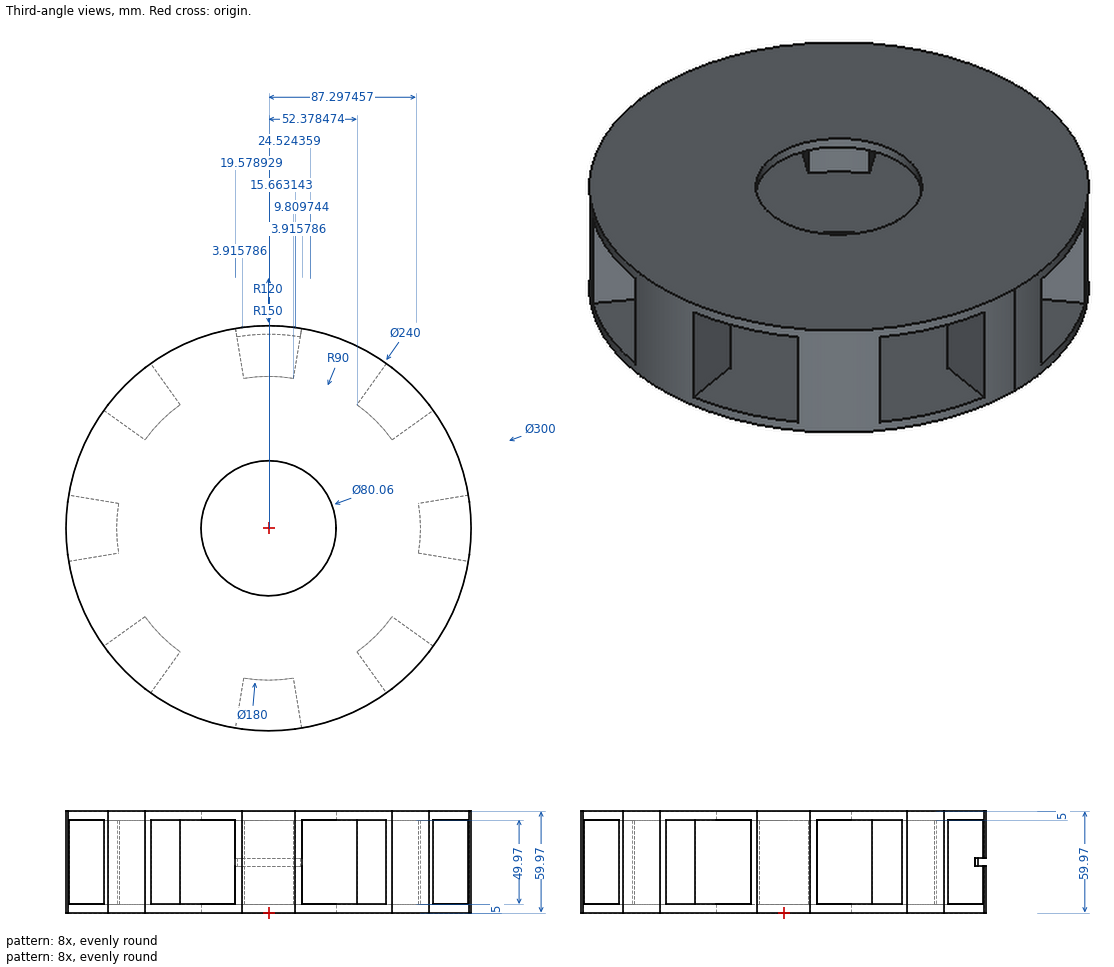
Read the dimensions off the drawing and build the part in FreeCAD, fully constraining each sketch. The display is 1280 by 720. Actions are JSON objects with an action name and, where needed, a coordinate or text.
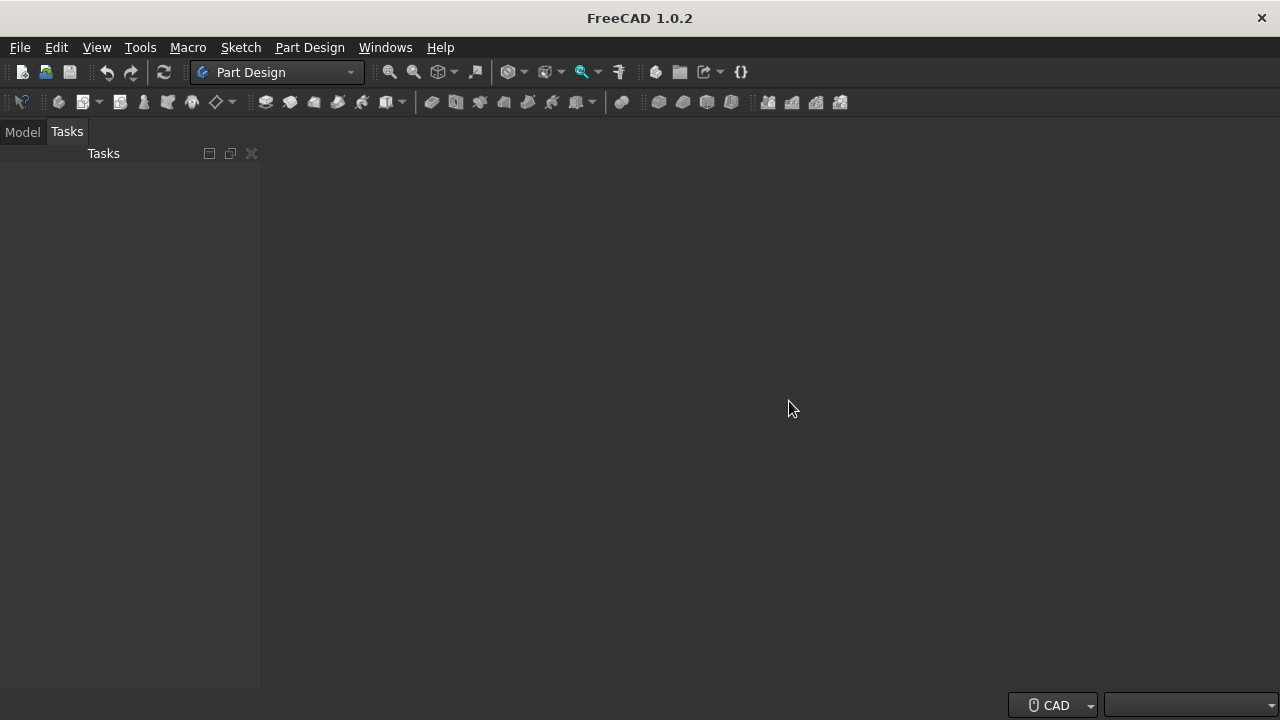
{"action": "left_click", "coordinate": [22, 72]}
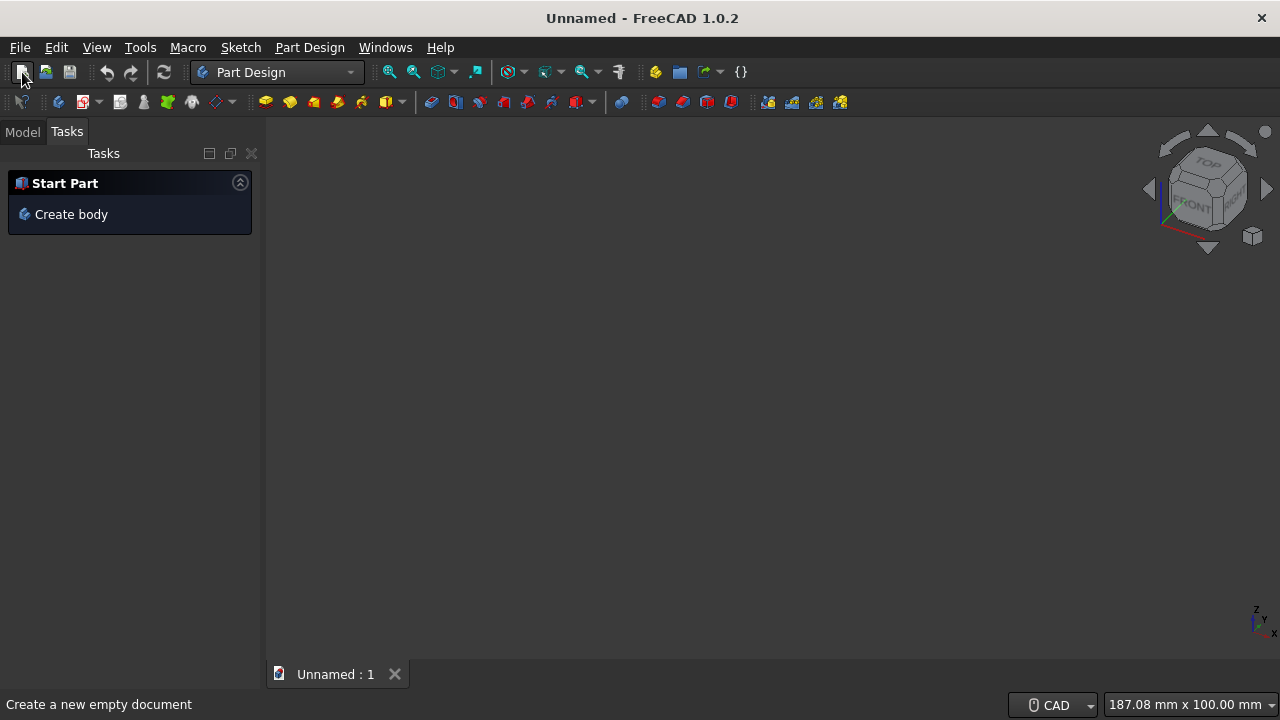
{"action": "left_click", "coordinate": [84, 102]}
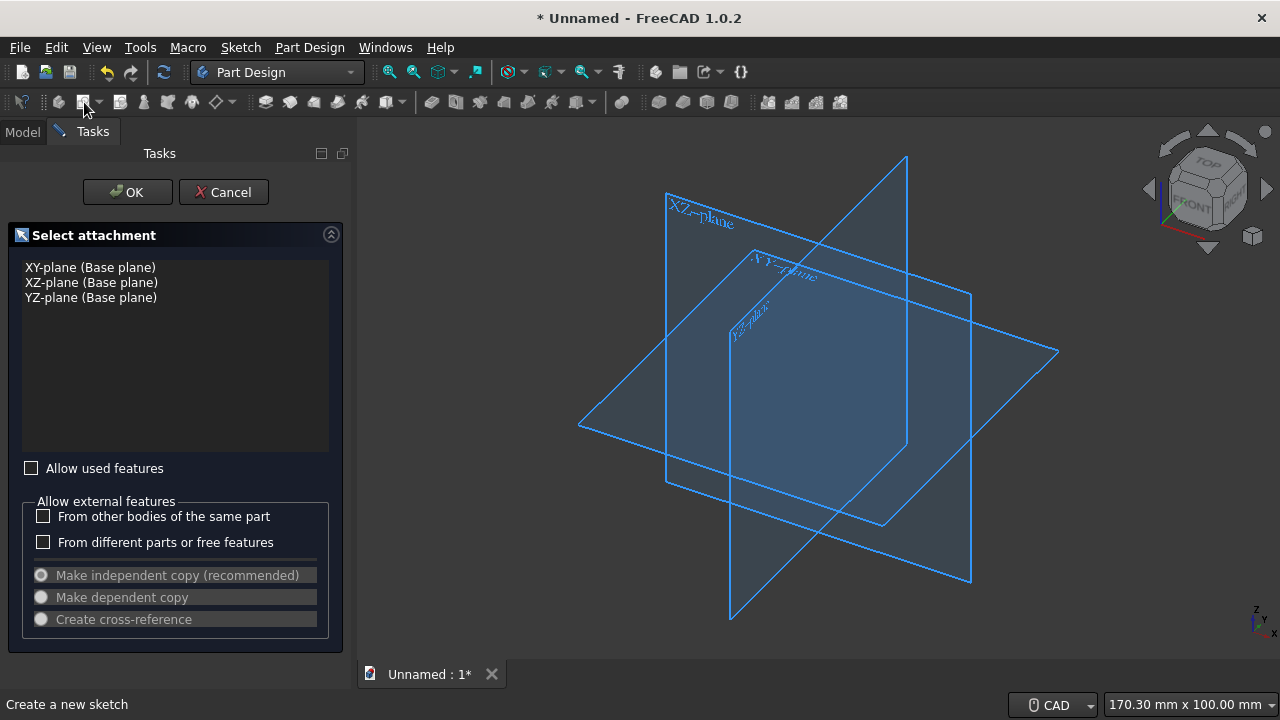
{"action": "left_click", "coordinate": [82, 268]}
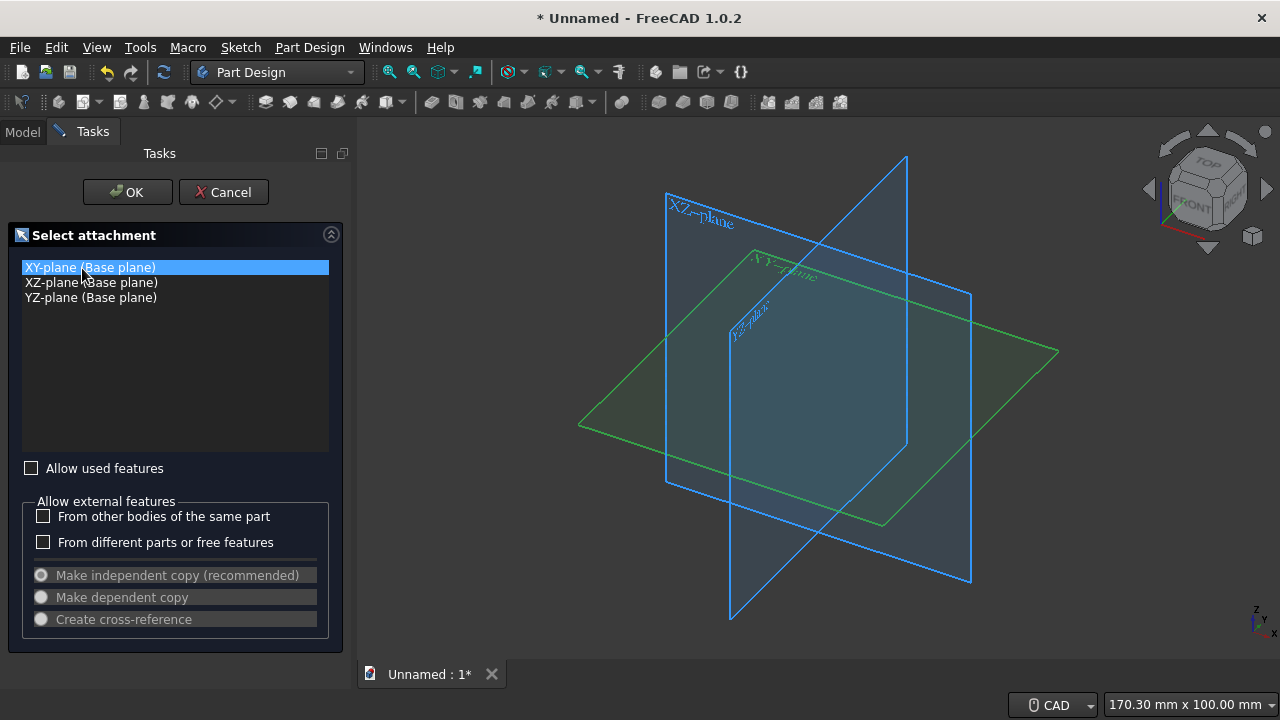
{"action": "left_click", "coordinate": [128, 192]}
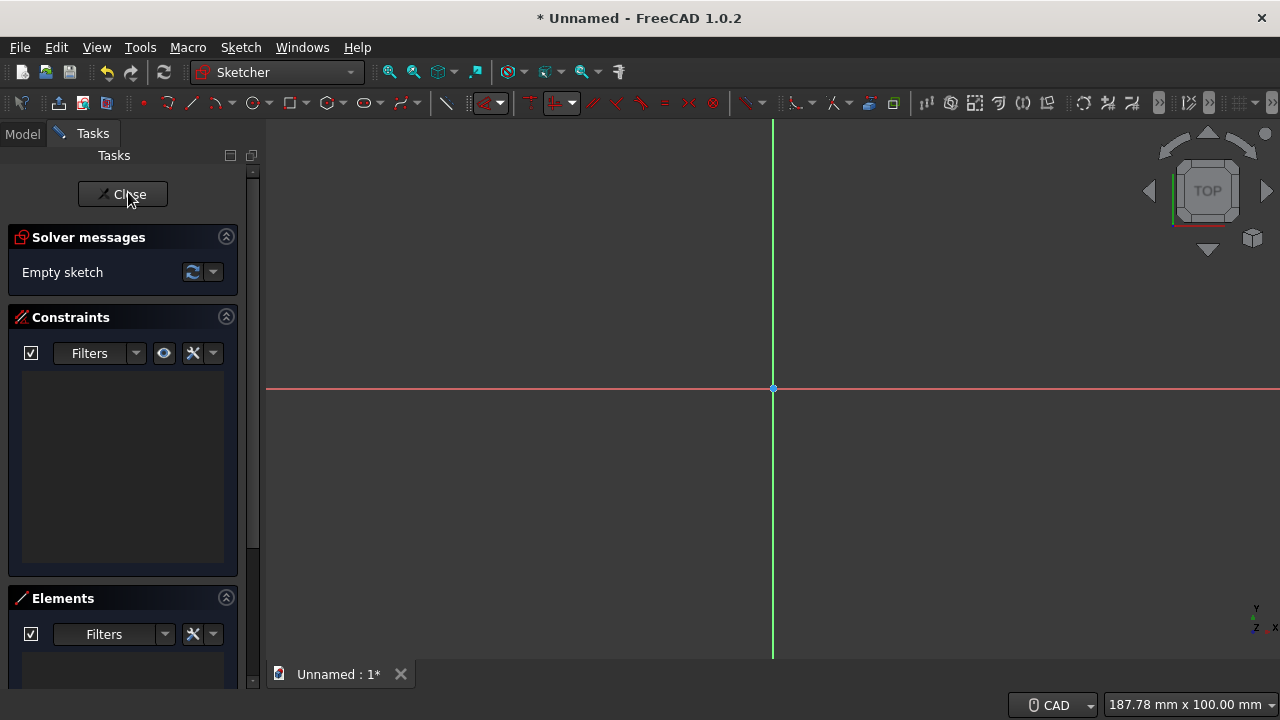
{"action": "scroll", "coordinate": [687, 389], "scroll_direction": "down", "scroll_amount": 8}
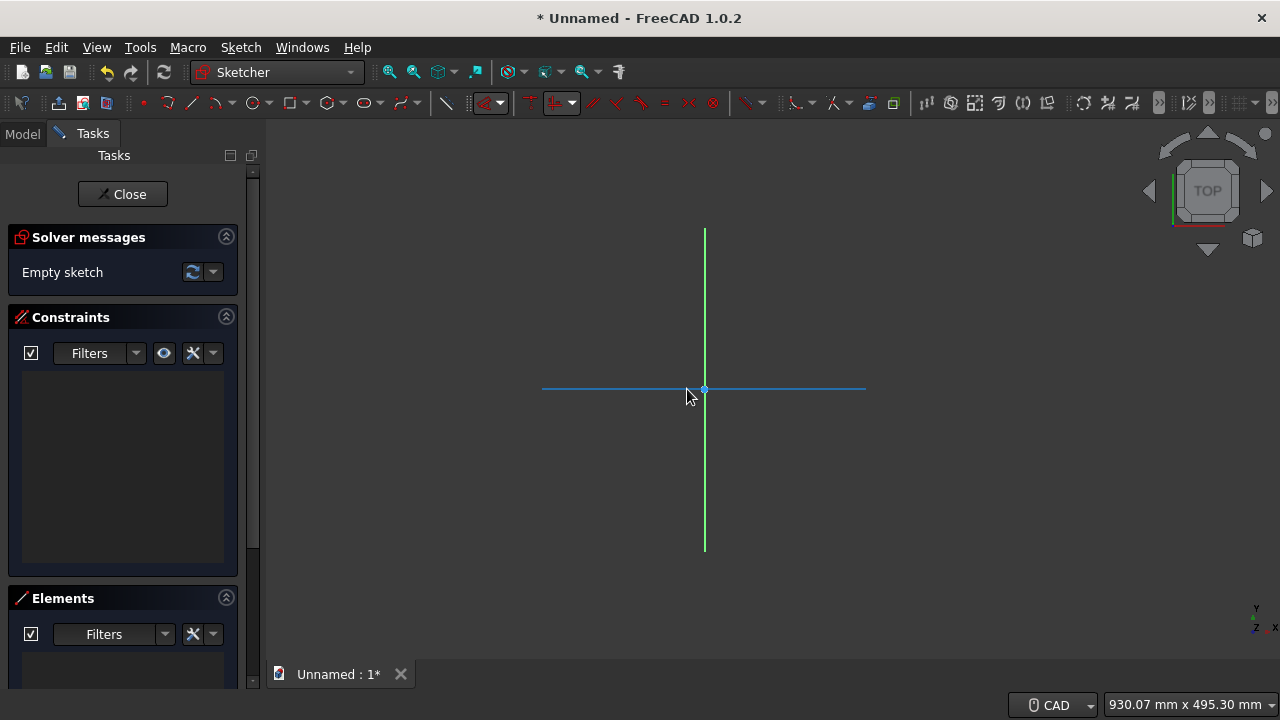
{"action": "left_click", "coordinate": [254, 104]}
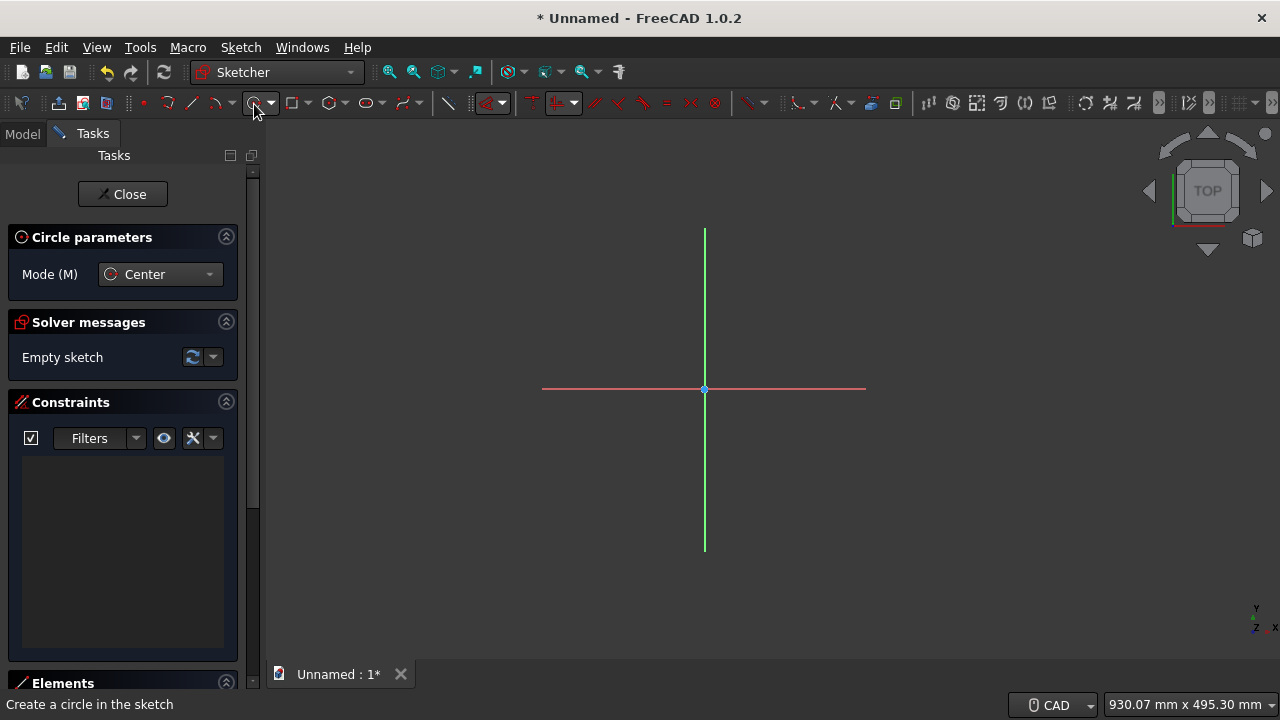
{"action": "left_click", "coordinate": [705, 389]}
{"action": "left_click", "coordinate": [820, 274]}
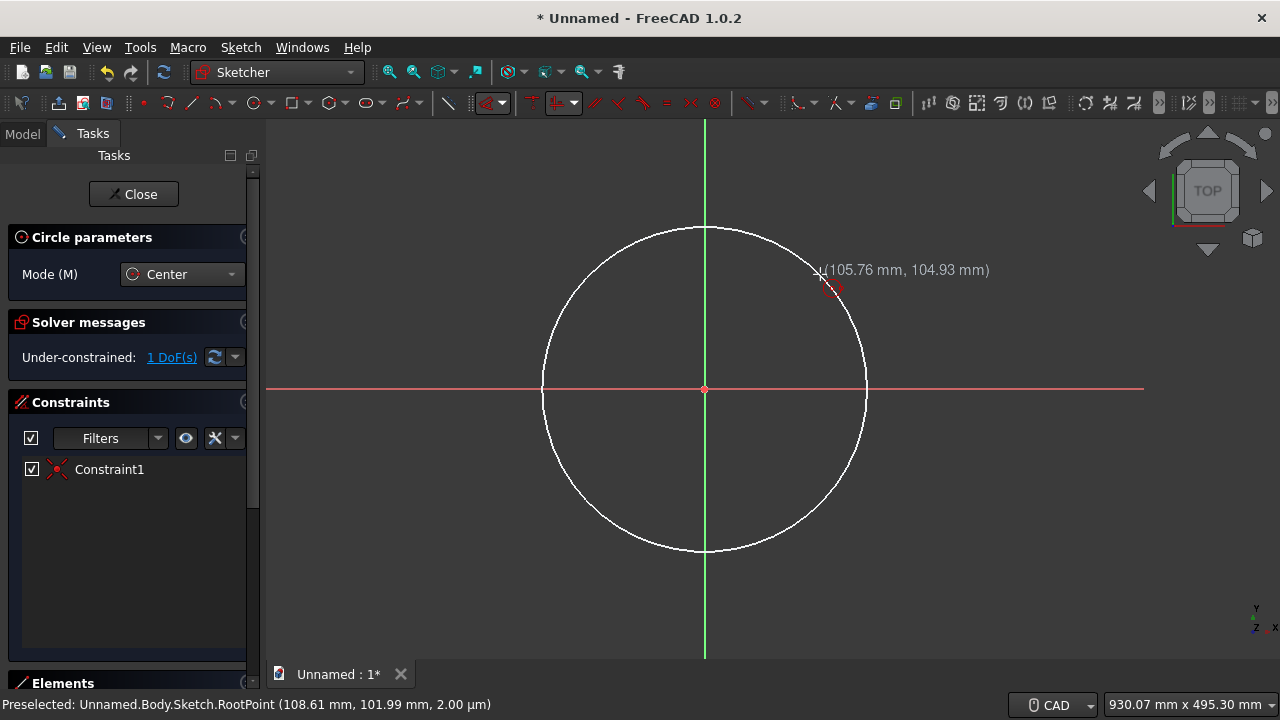
{"action": "left_click", "coordinate": [705, 389]}
{"action": "left_click", "coordinate": [797, 297]}
{"action": "key", "text": "Escape"}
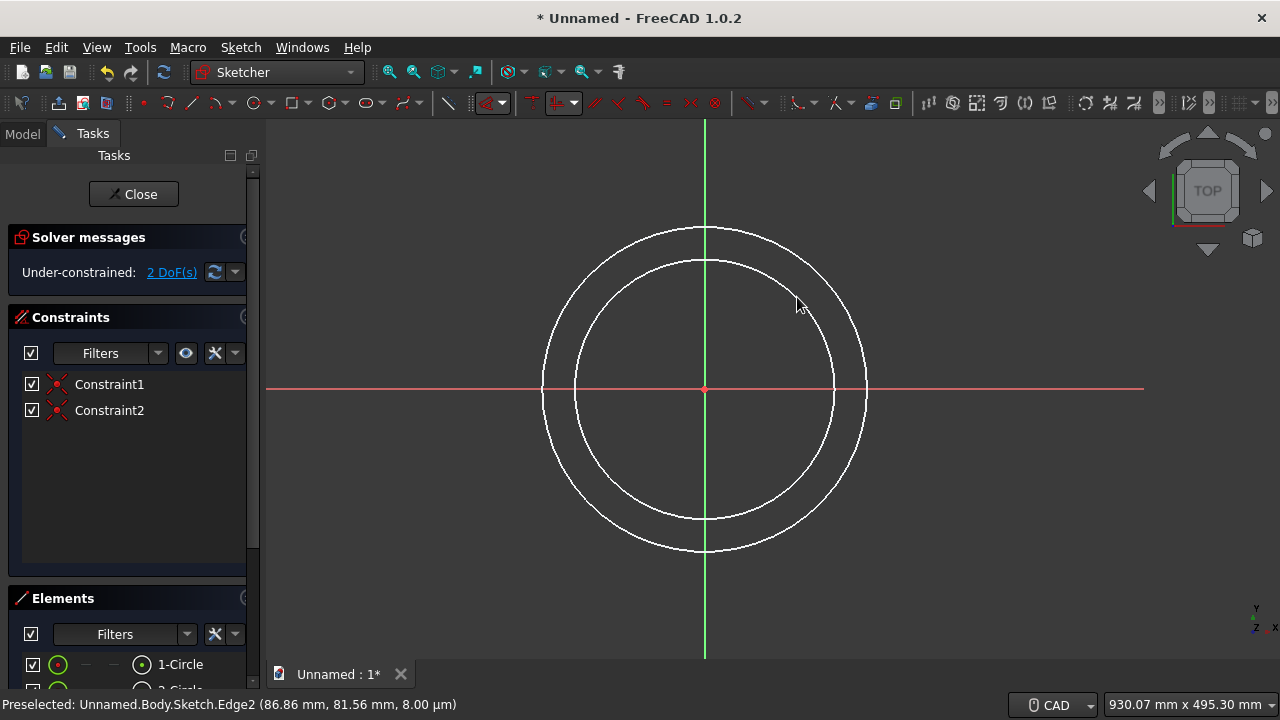
{"action": "key", "text": "d"}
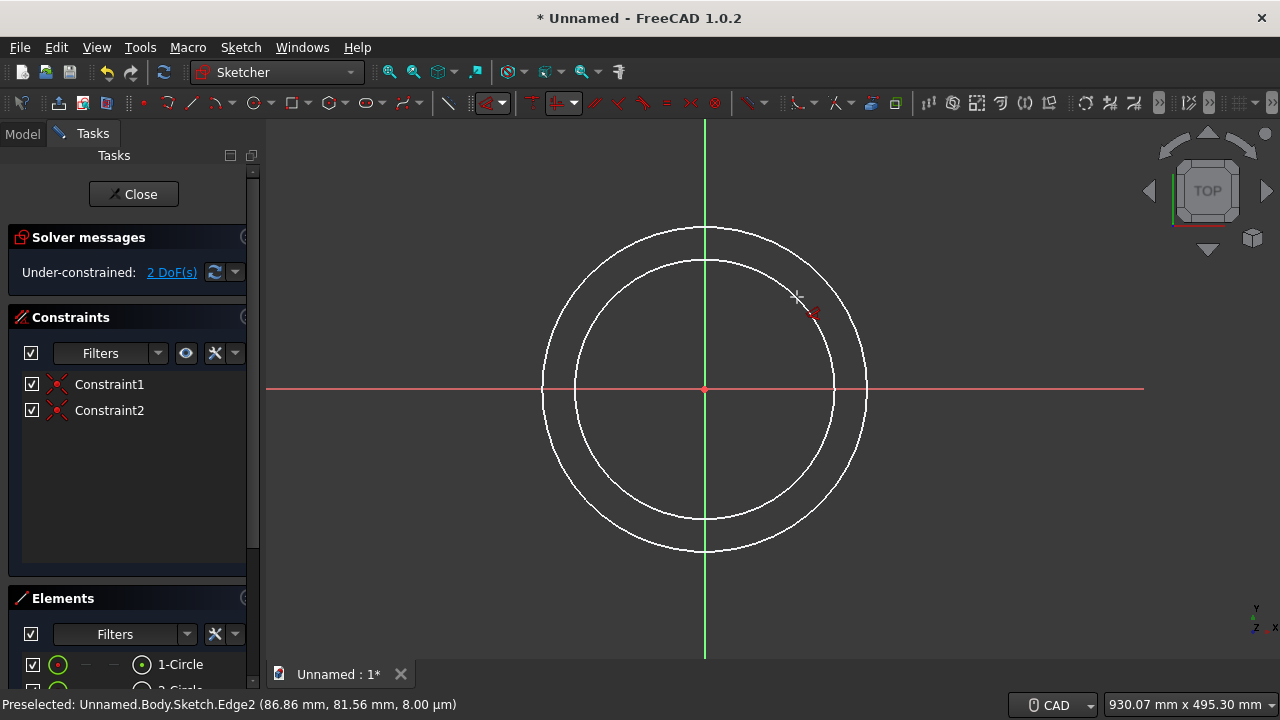
{"action": "left_click", "coordinate": [819, 274]}
{"action": "left_click", "coordinate": [842, 251]}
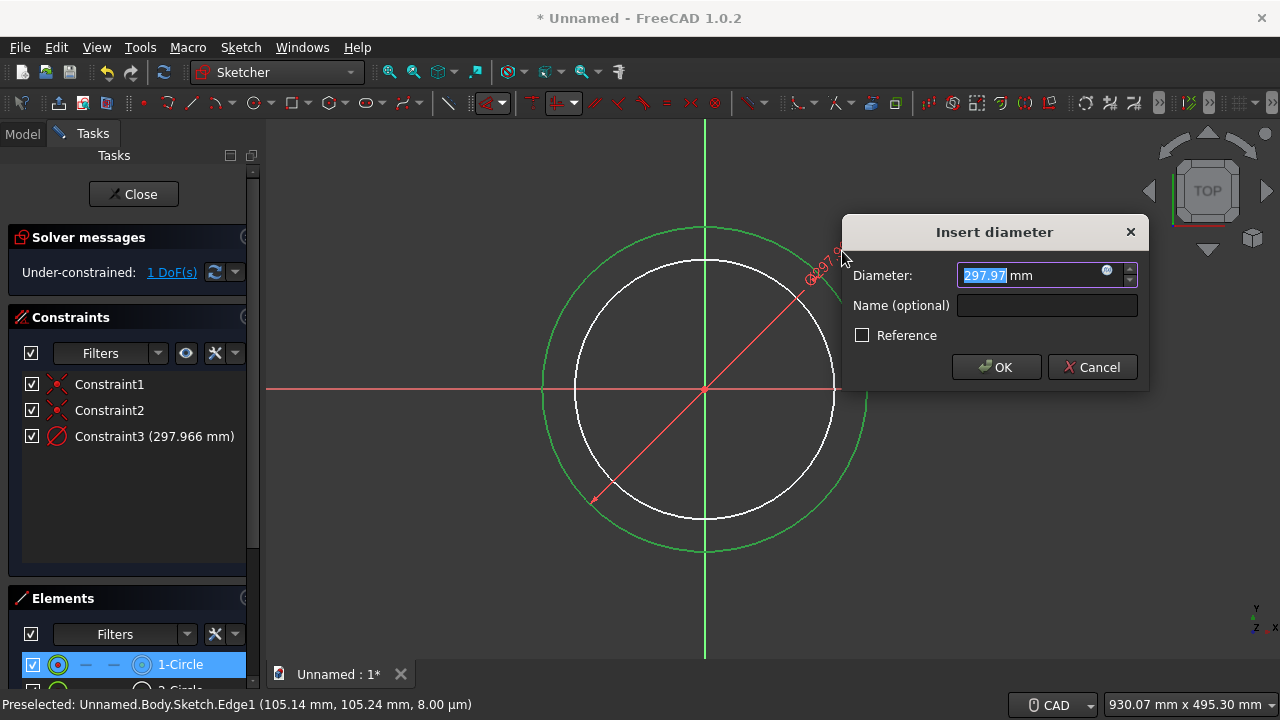
{"action": "type", "text": "300"}
{"action": "key", "text": "Return"}